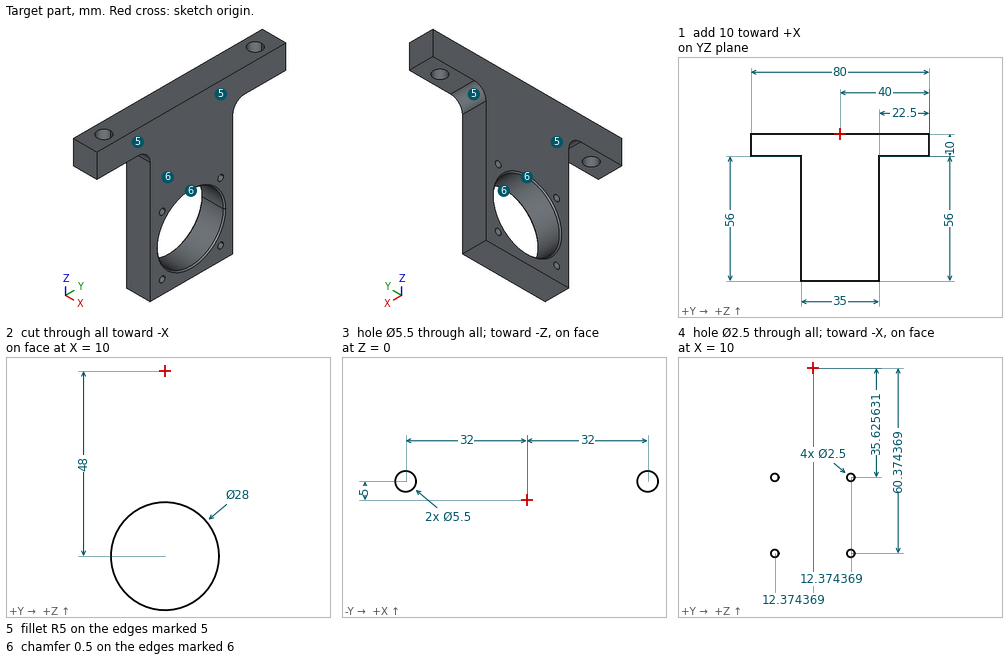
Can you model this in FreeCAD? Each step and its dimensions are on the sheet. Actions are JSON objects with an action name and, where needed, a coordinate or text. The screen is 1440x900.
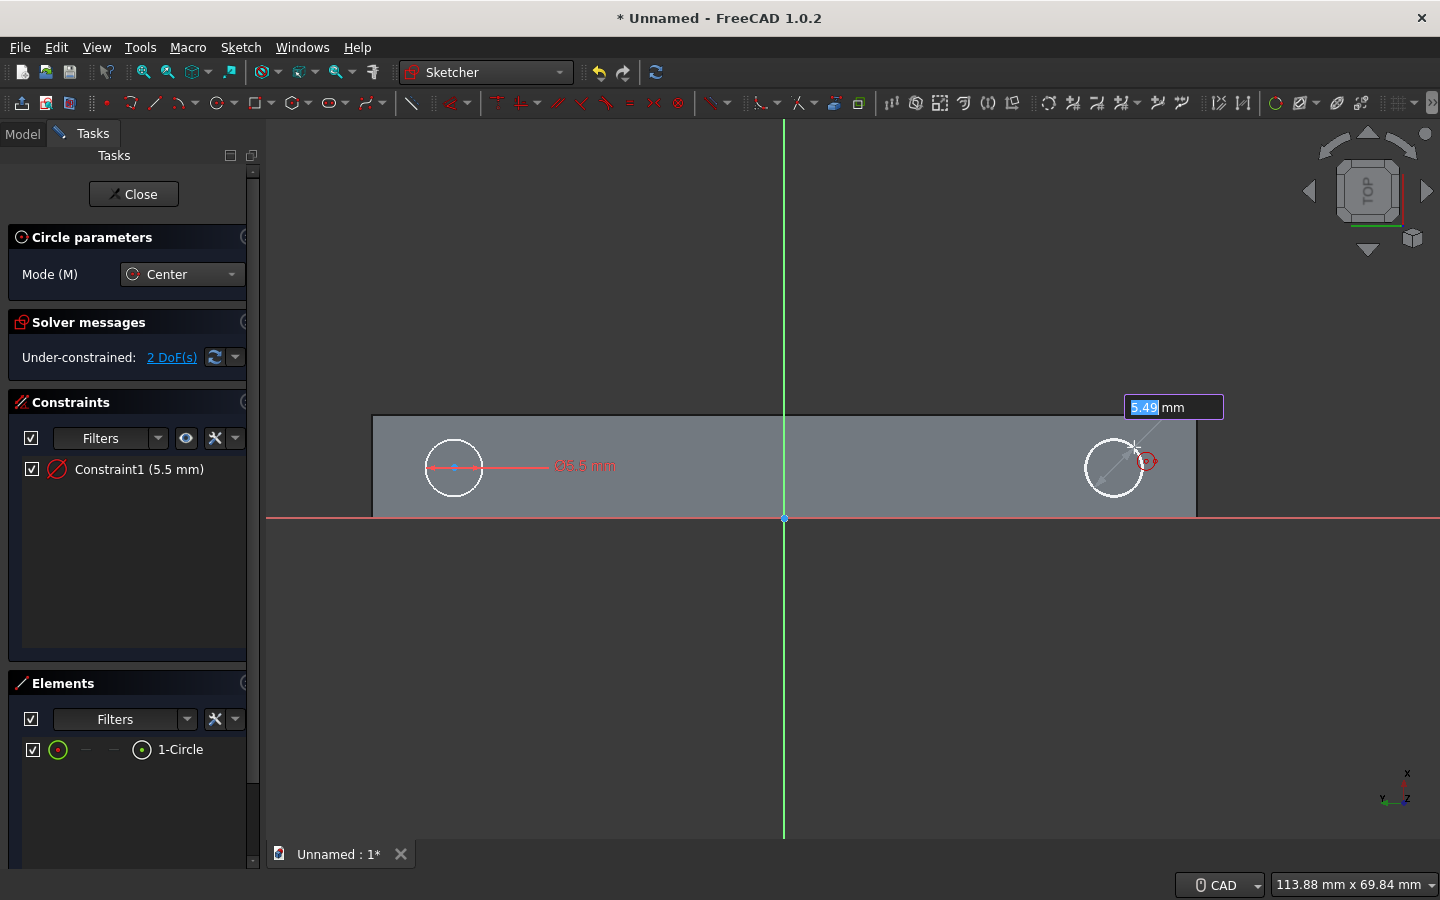
{"action": "type", "text": "5.5"}
{"action": "key", "text": "Return"}
{"action": "key", "text": "Escape"}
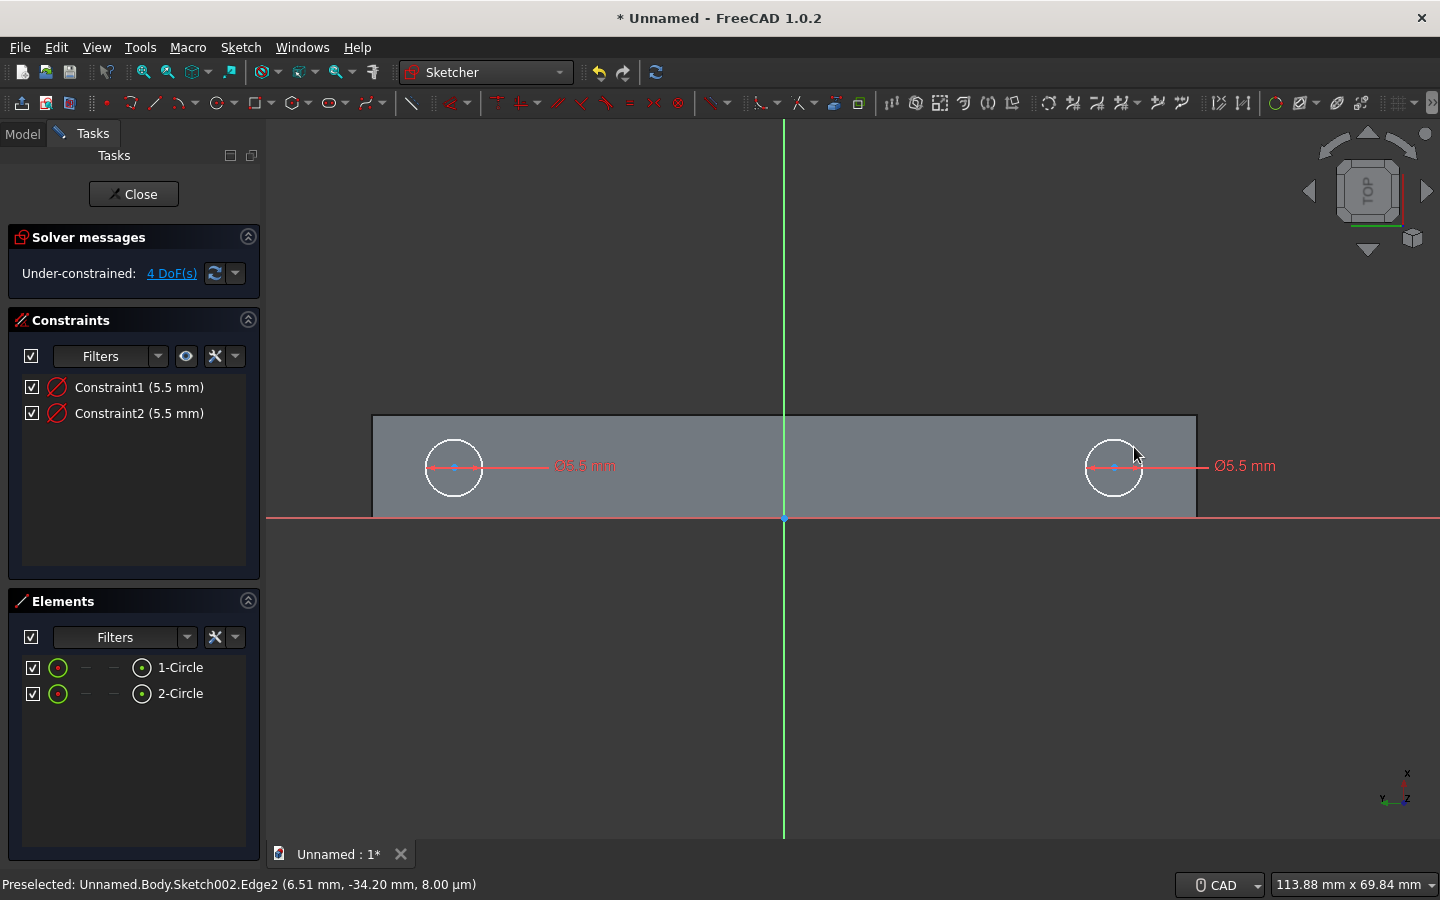
{"action": "left_click", "coordinate": [454, 468]}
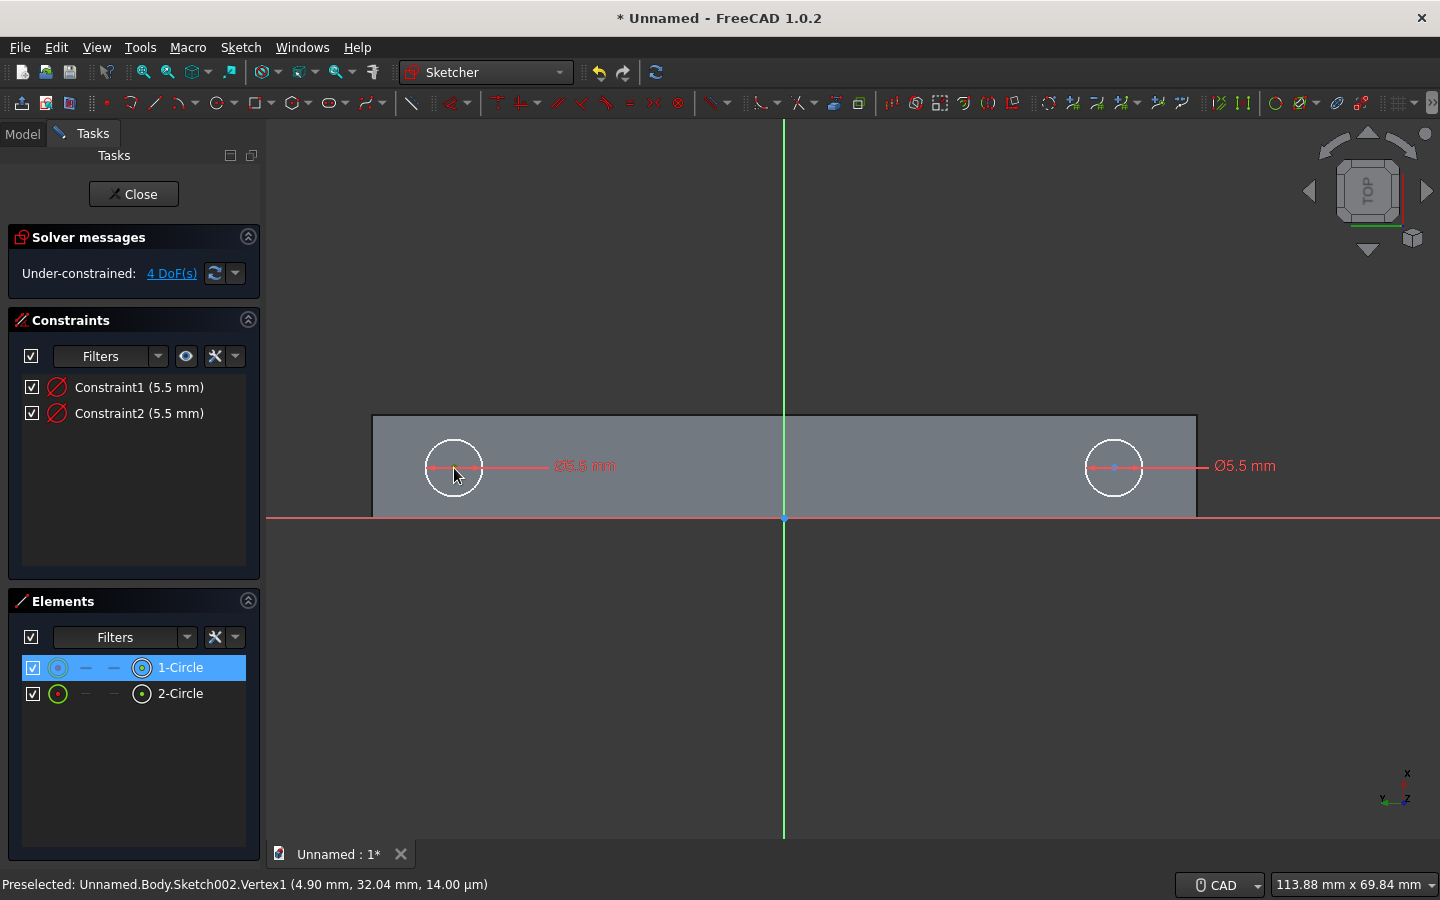
{"action": "left_click", "coordinate": [1114, 468]}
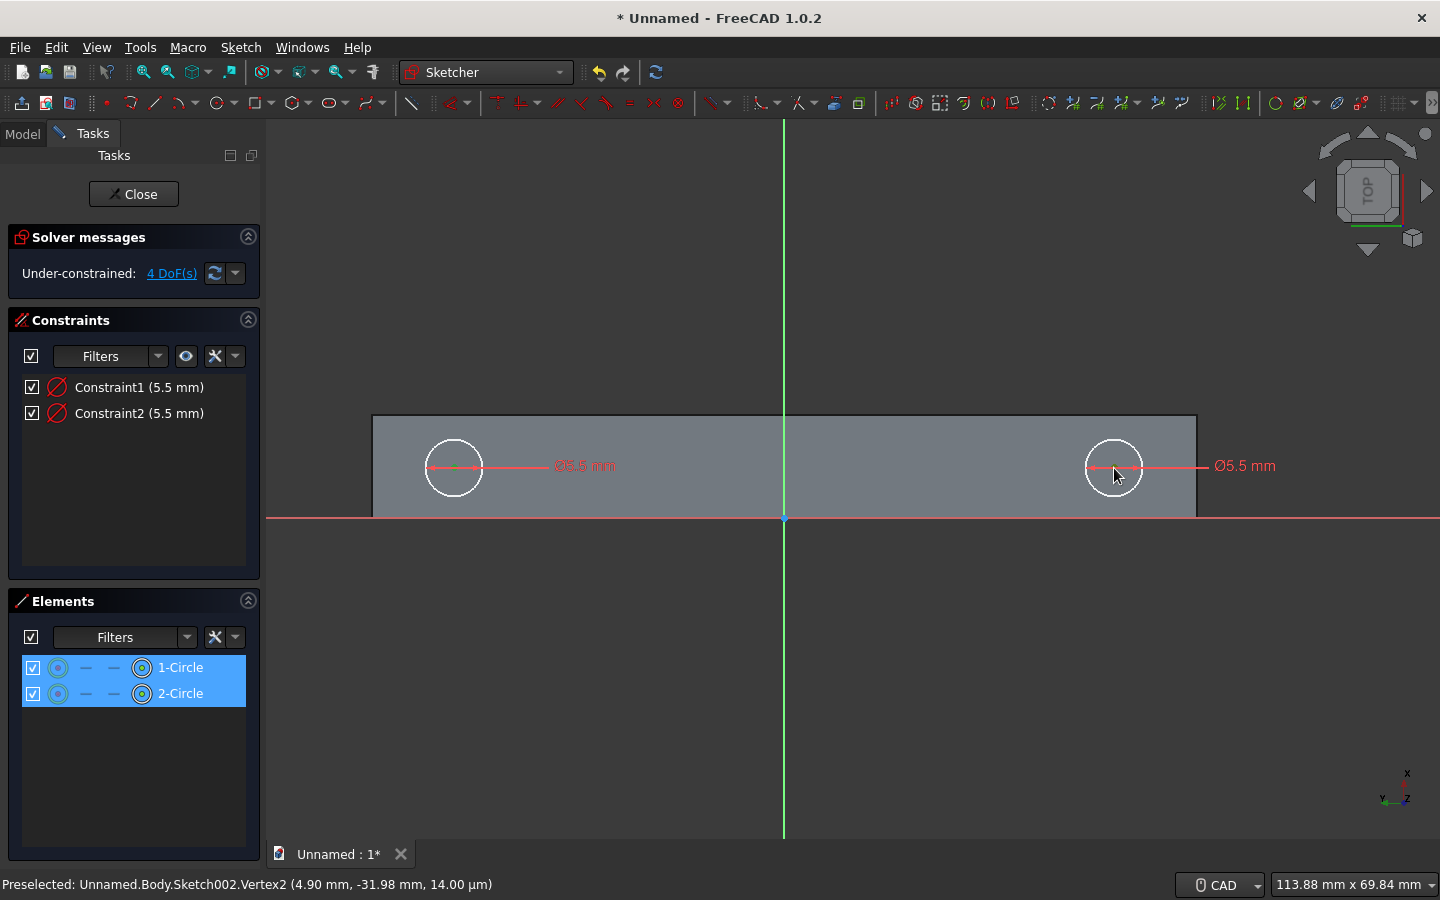
{"action": "left_click", "coordinate": [540, 104]}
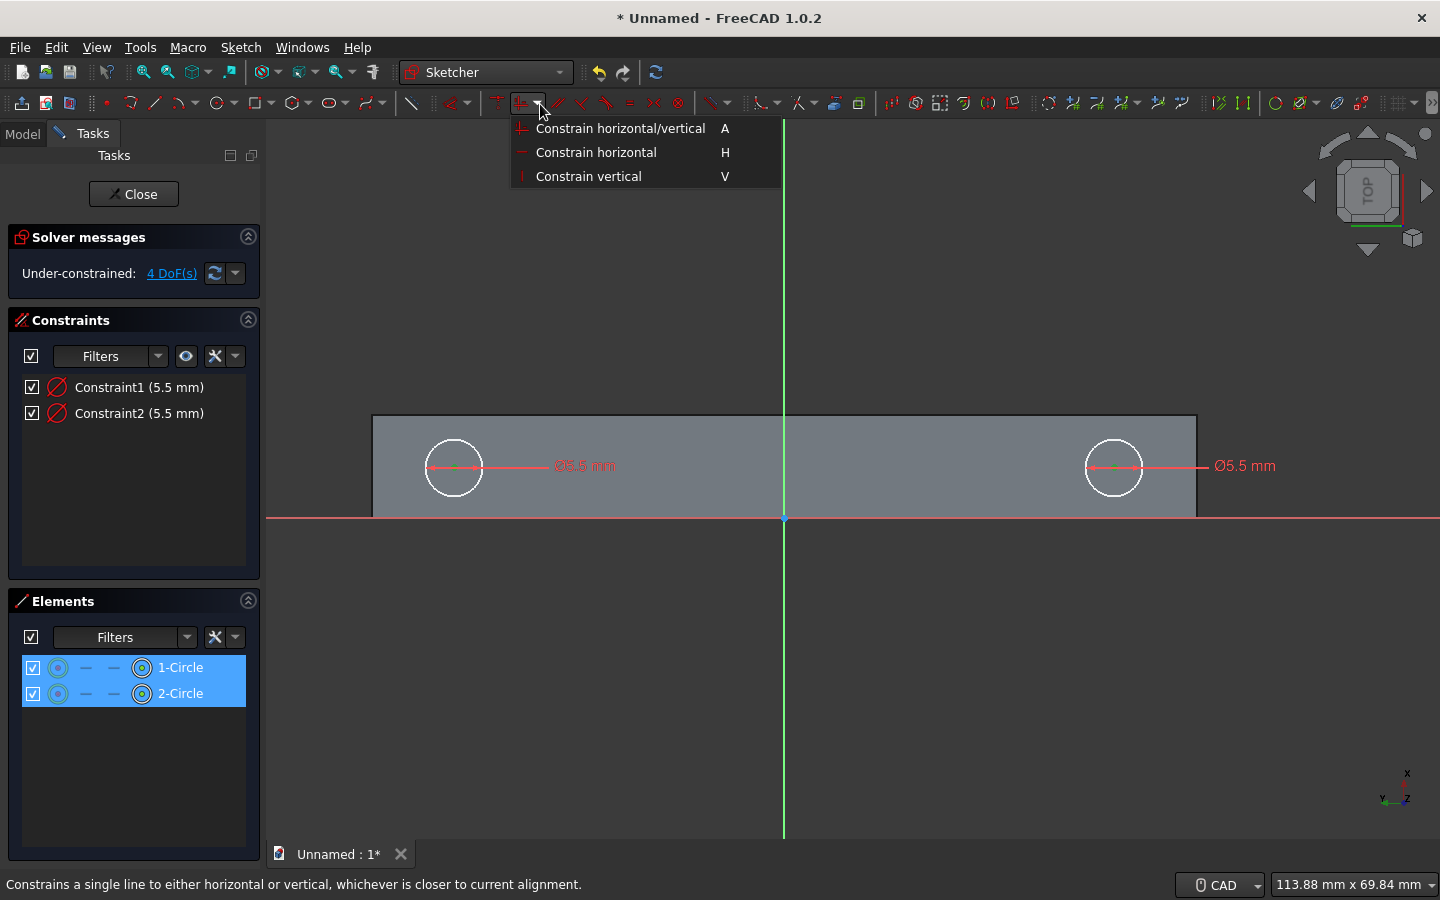
{"action": "left_click", "coordinate": [646, 152]}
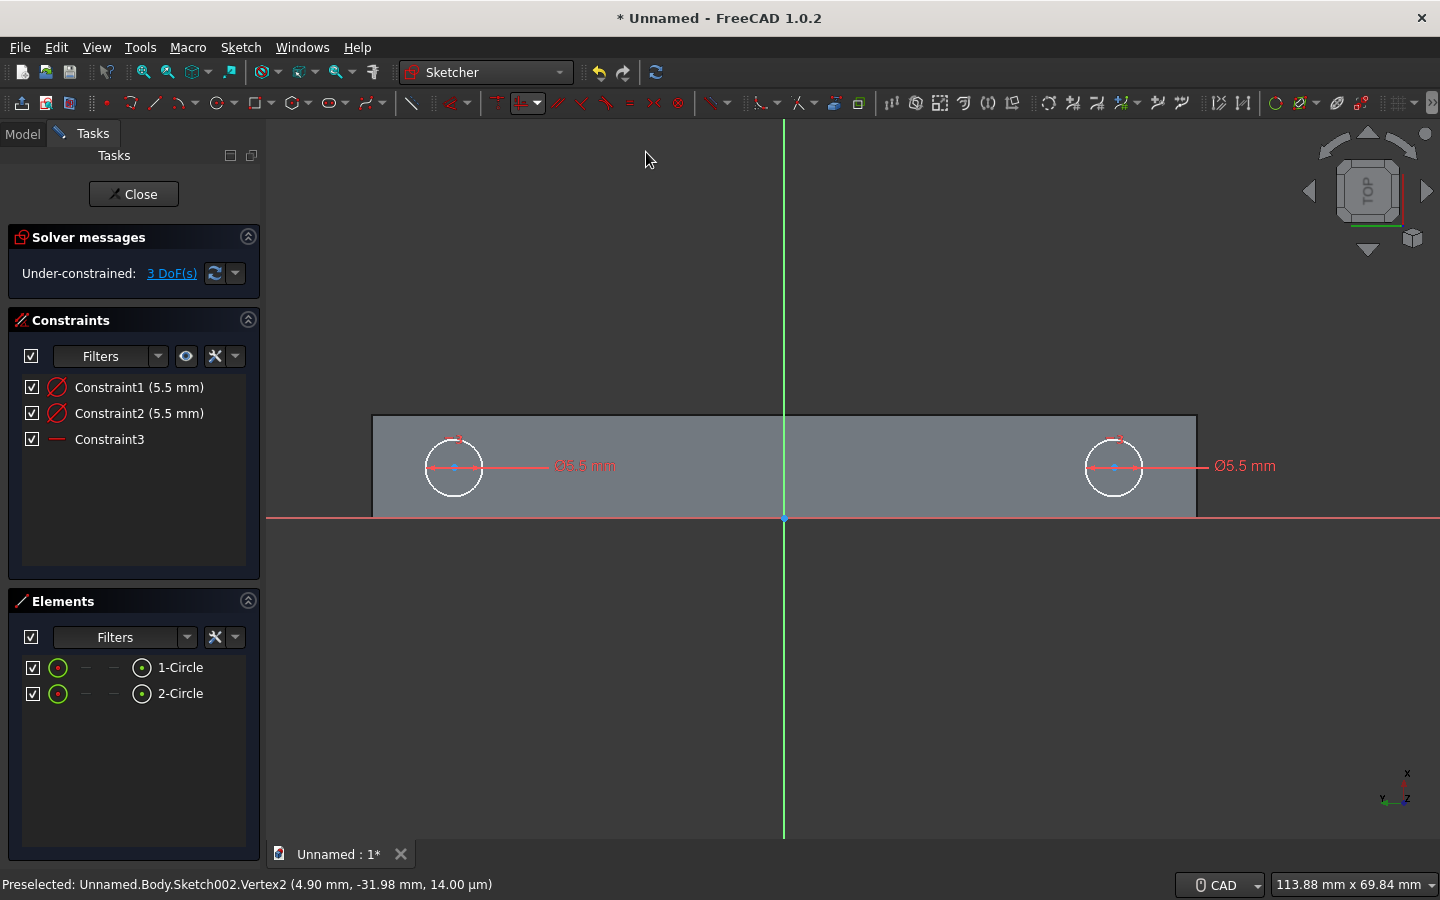
{"action": "left_click", "coordinate": [450, 104]}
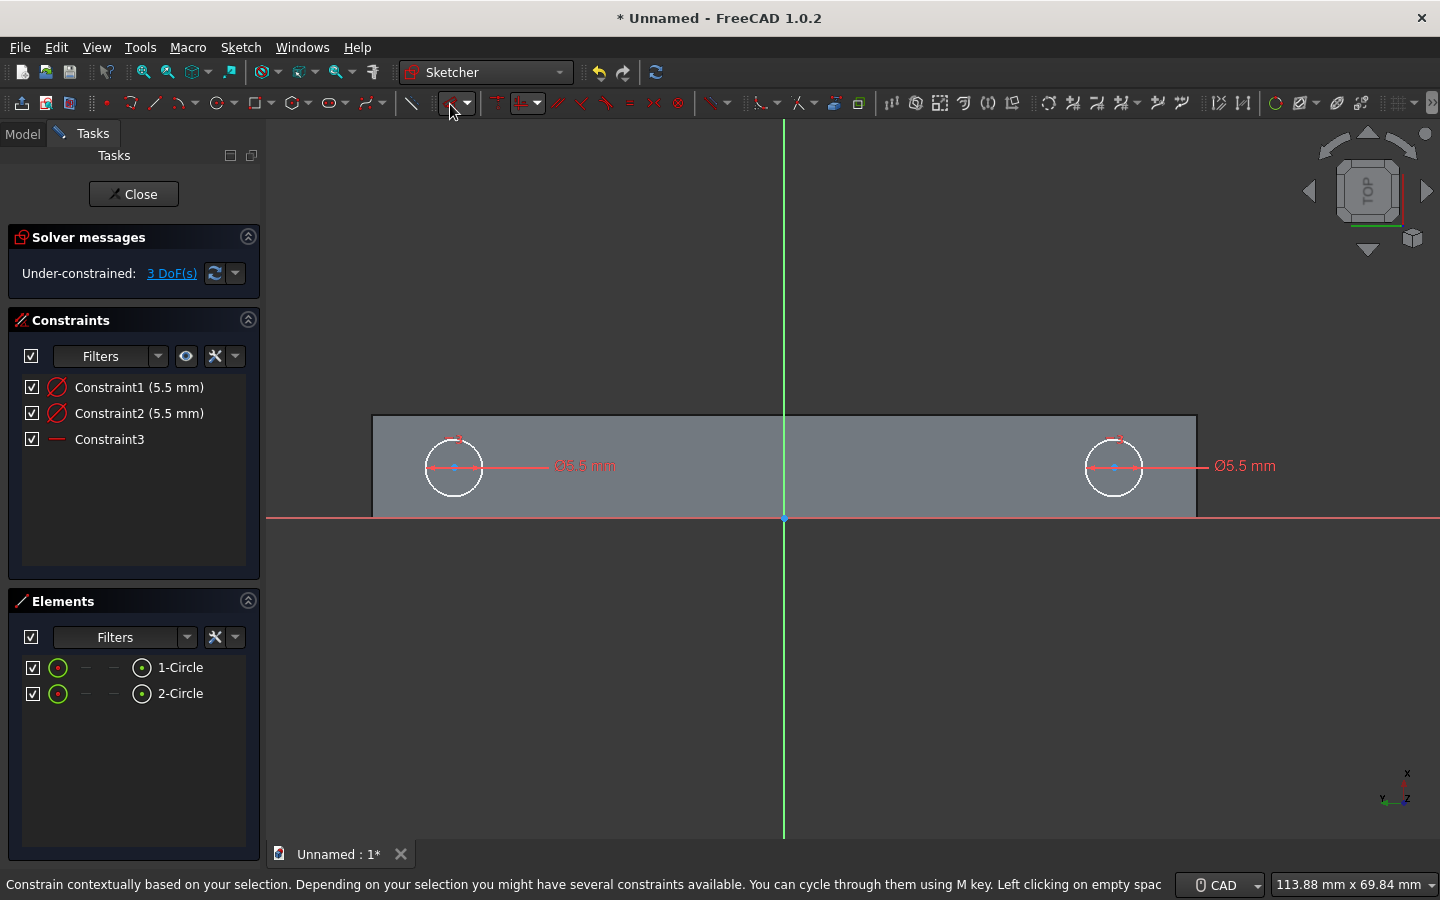
{"action": "left_click", "coordinate": [454, 468]}
{"action": "left_click", "coordinate": [420, 493]}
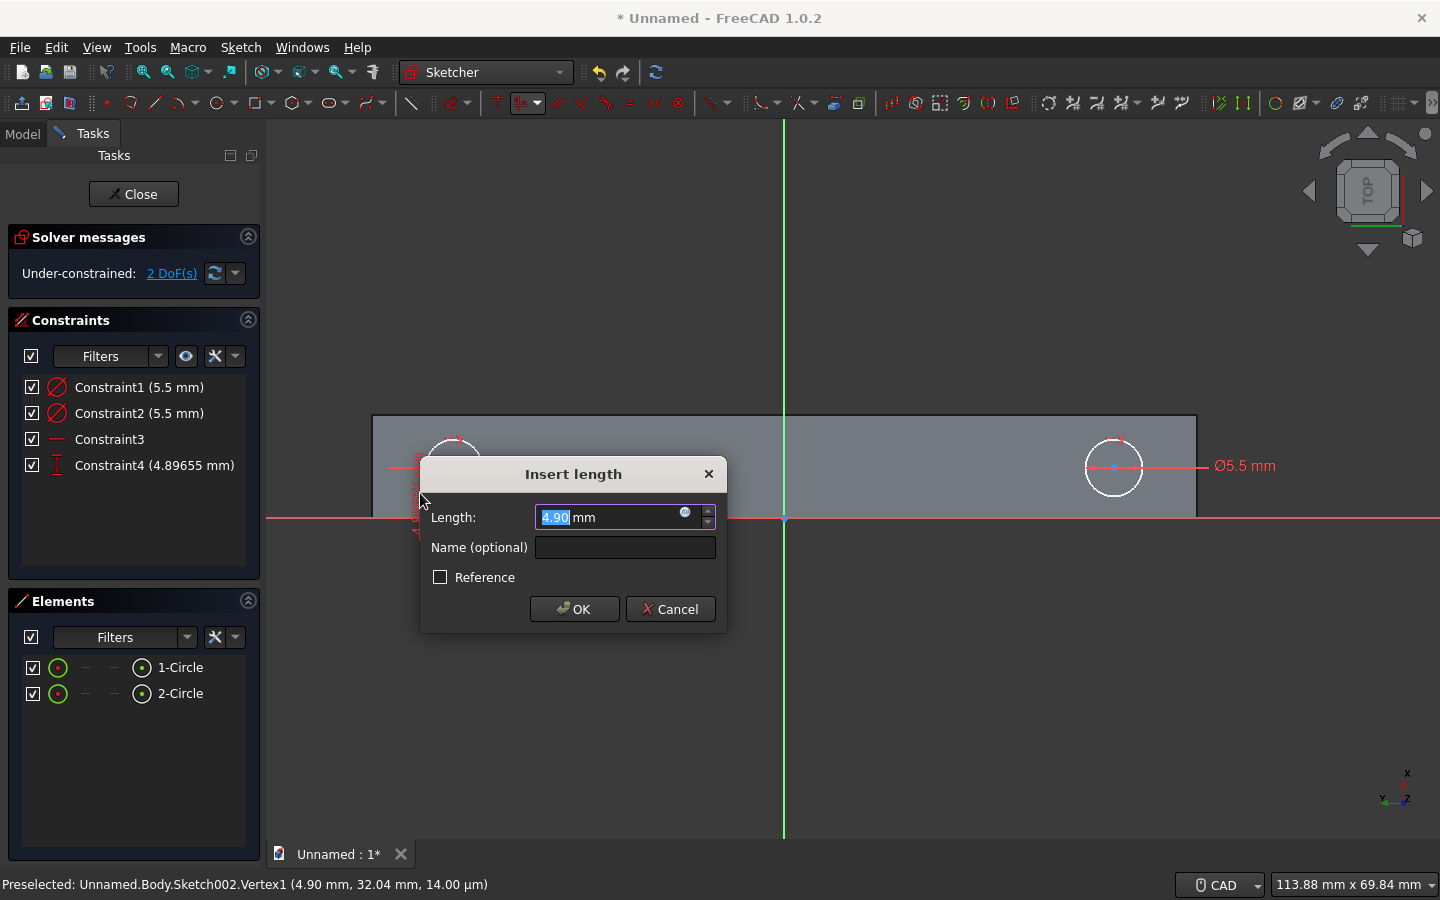
{"action": "type", "text": "5"}
{"action": "key", "text": "Return"}